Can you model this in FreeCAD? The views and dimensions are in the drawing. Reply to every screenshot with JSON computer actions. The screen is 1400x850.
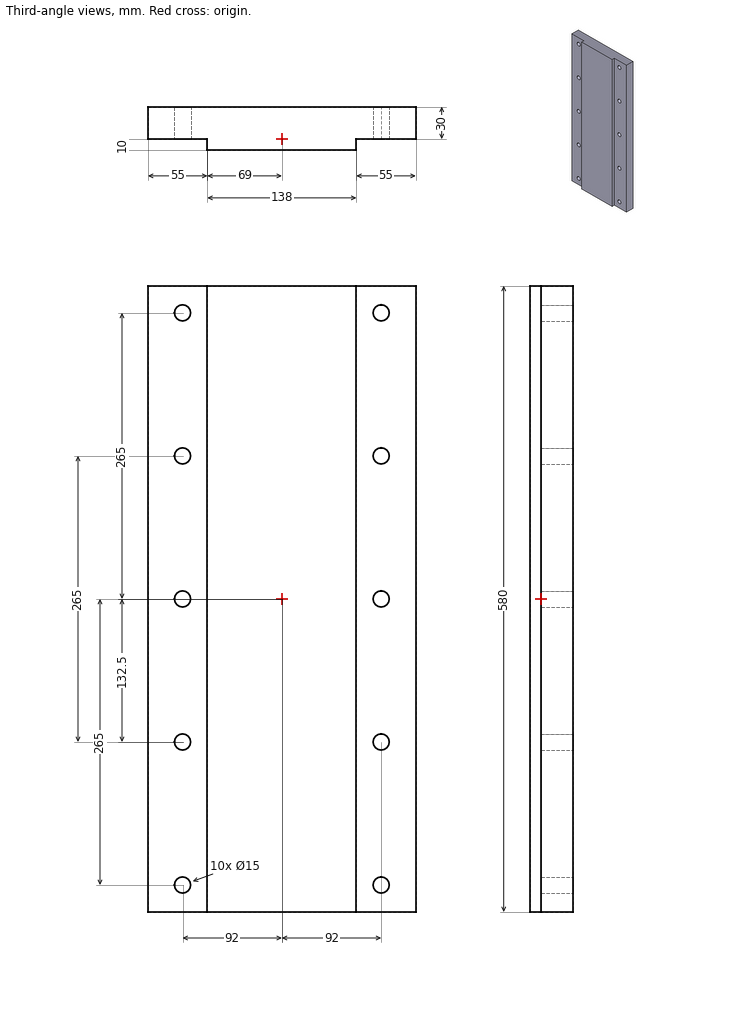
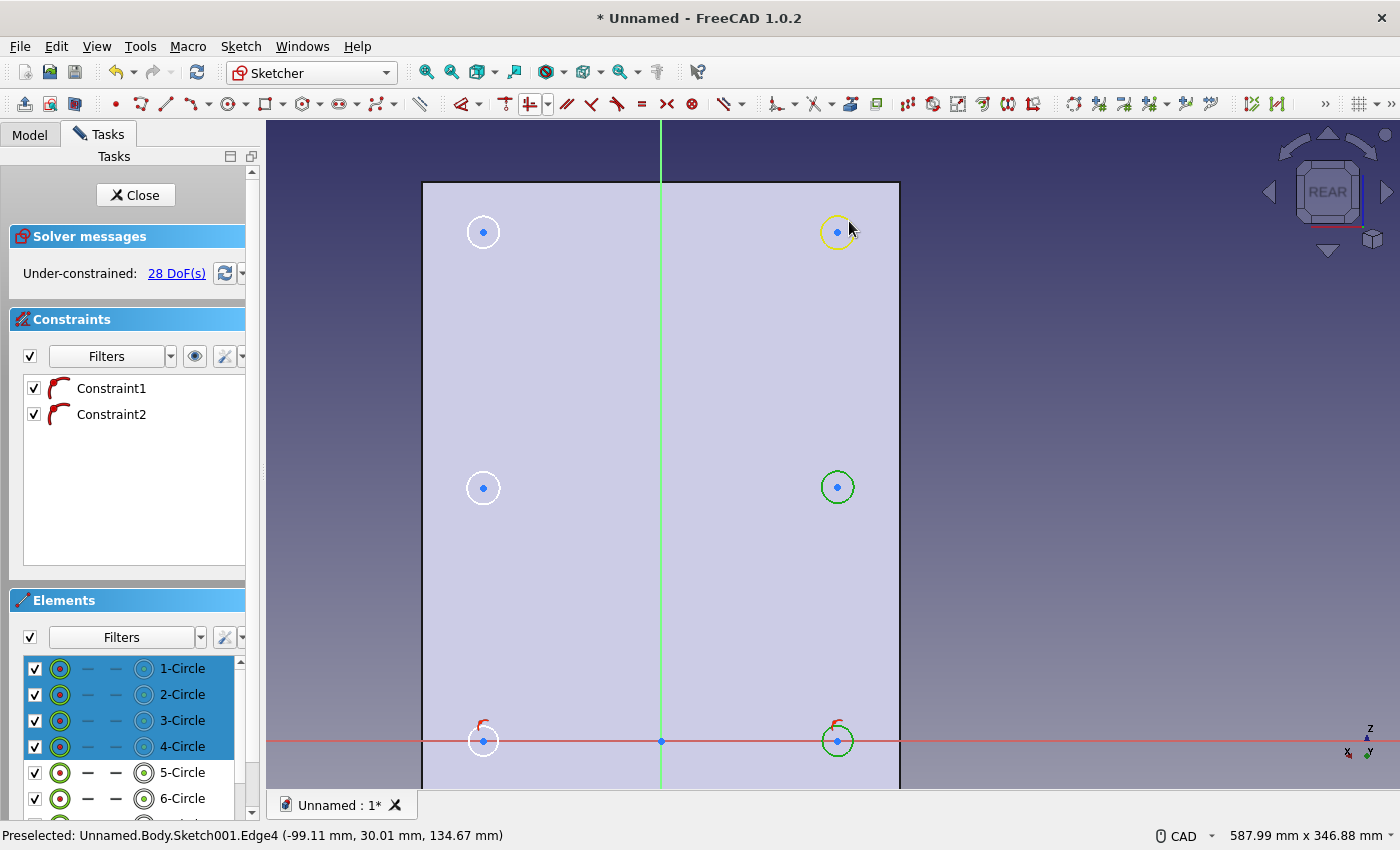
{"action": "left_click", "coordinate": [849, 221]}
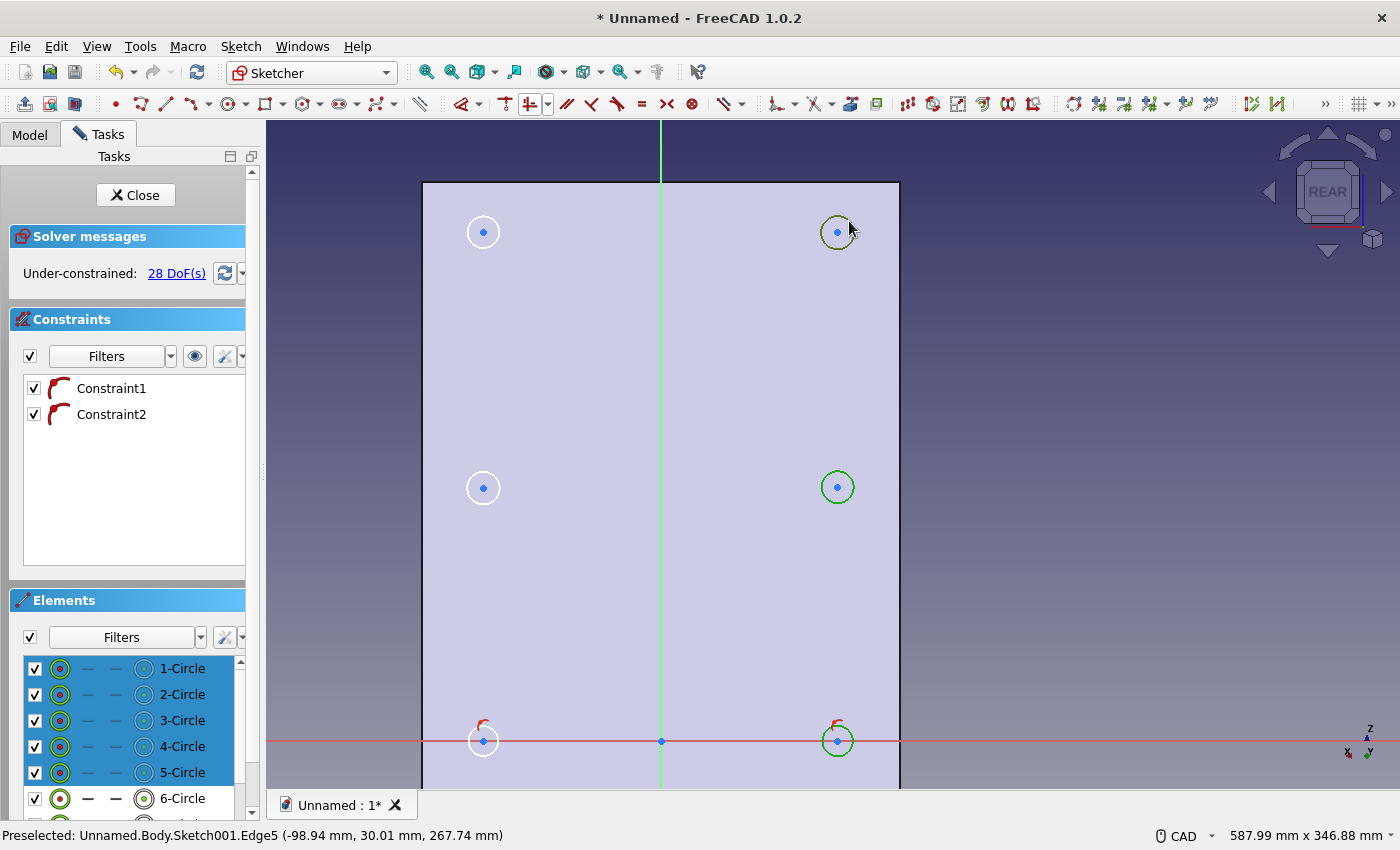
{"action": "scroll", "coordinate": [849, 221], "scroll_direction": "down", "scroll_amount": 4}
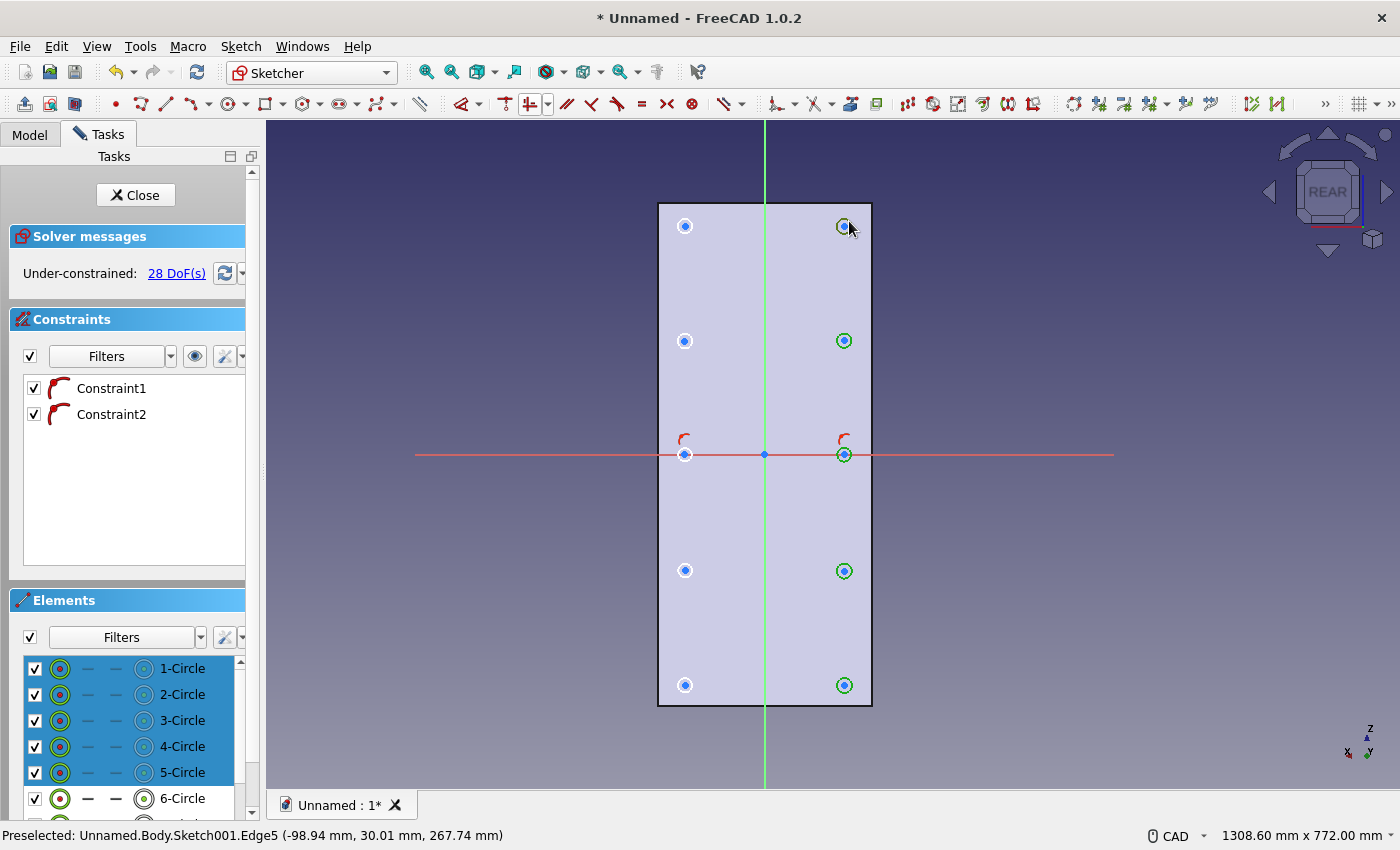
{"action": "scroll", "coordinate": [690, 566], "scroll_direction": "up", "scroll_amount": 4}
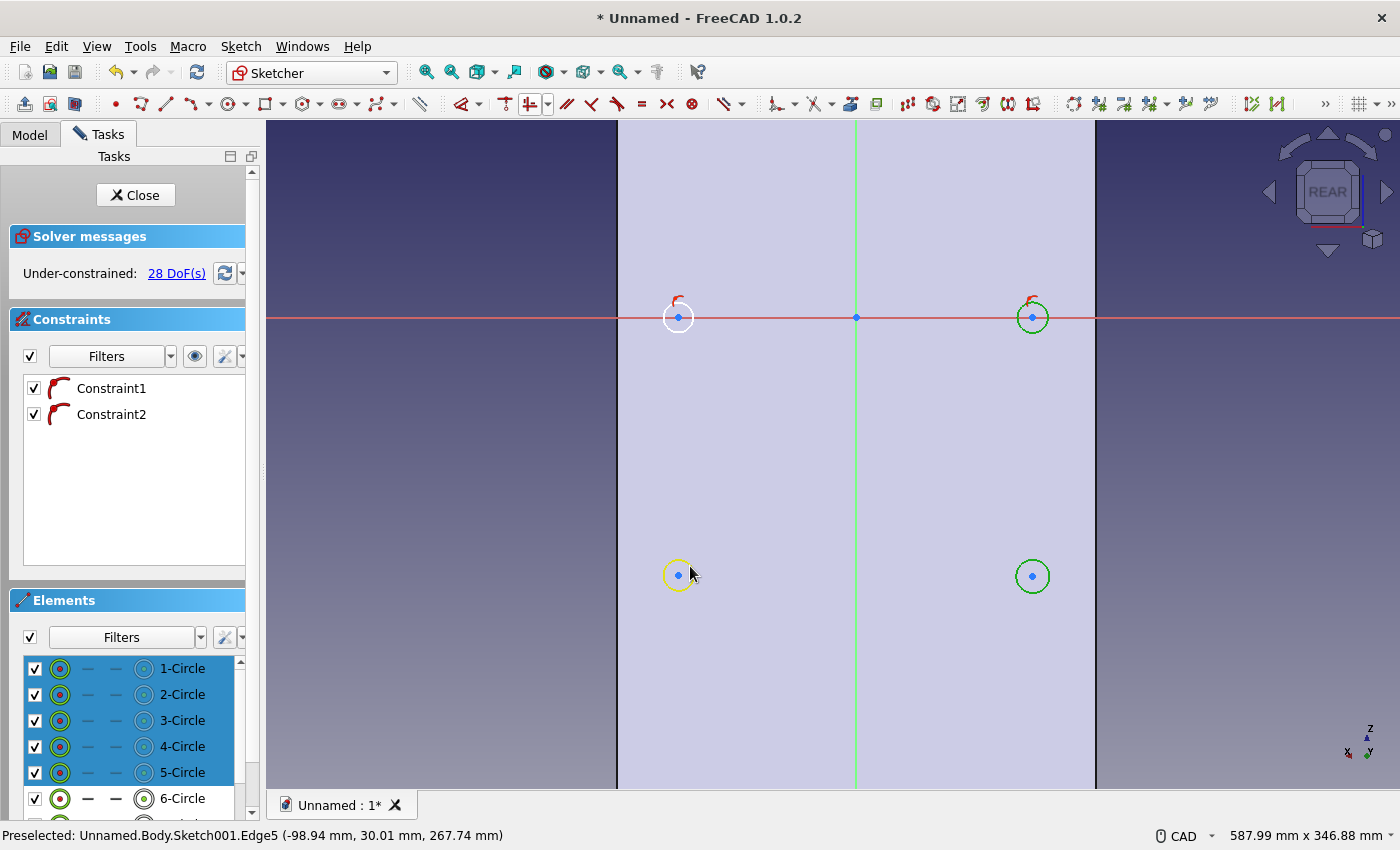
{"action": "left_click", "coordinate": [690, 565]}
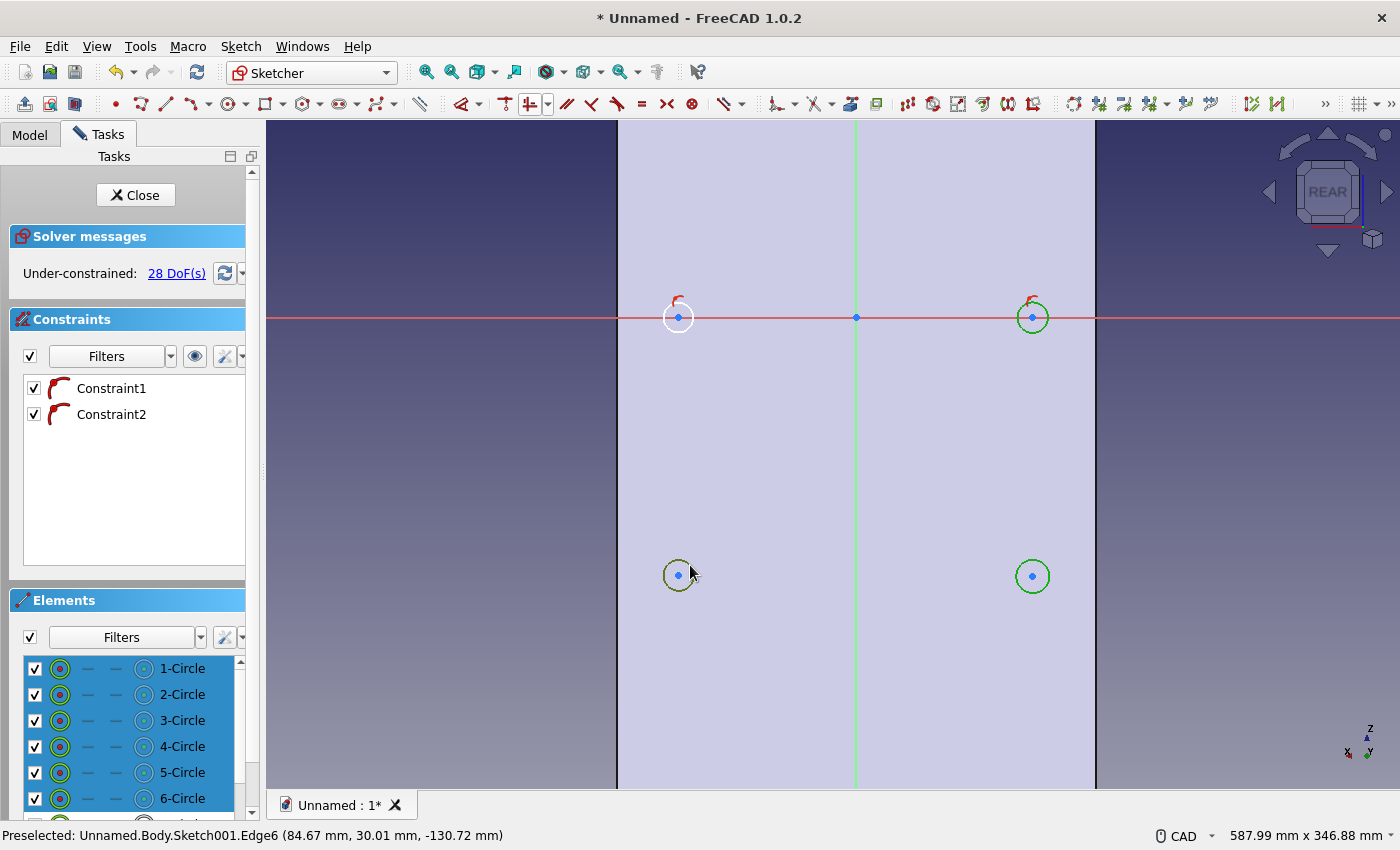
{"action": "scroll", "coordinate": [689, 307], "scroll_direction": "up", "scroll_amount": 2}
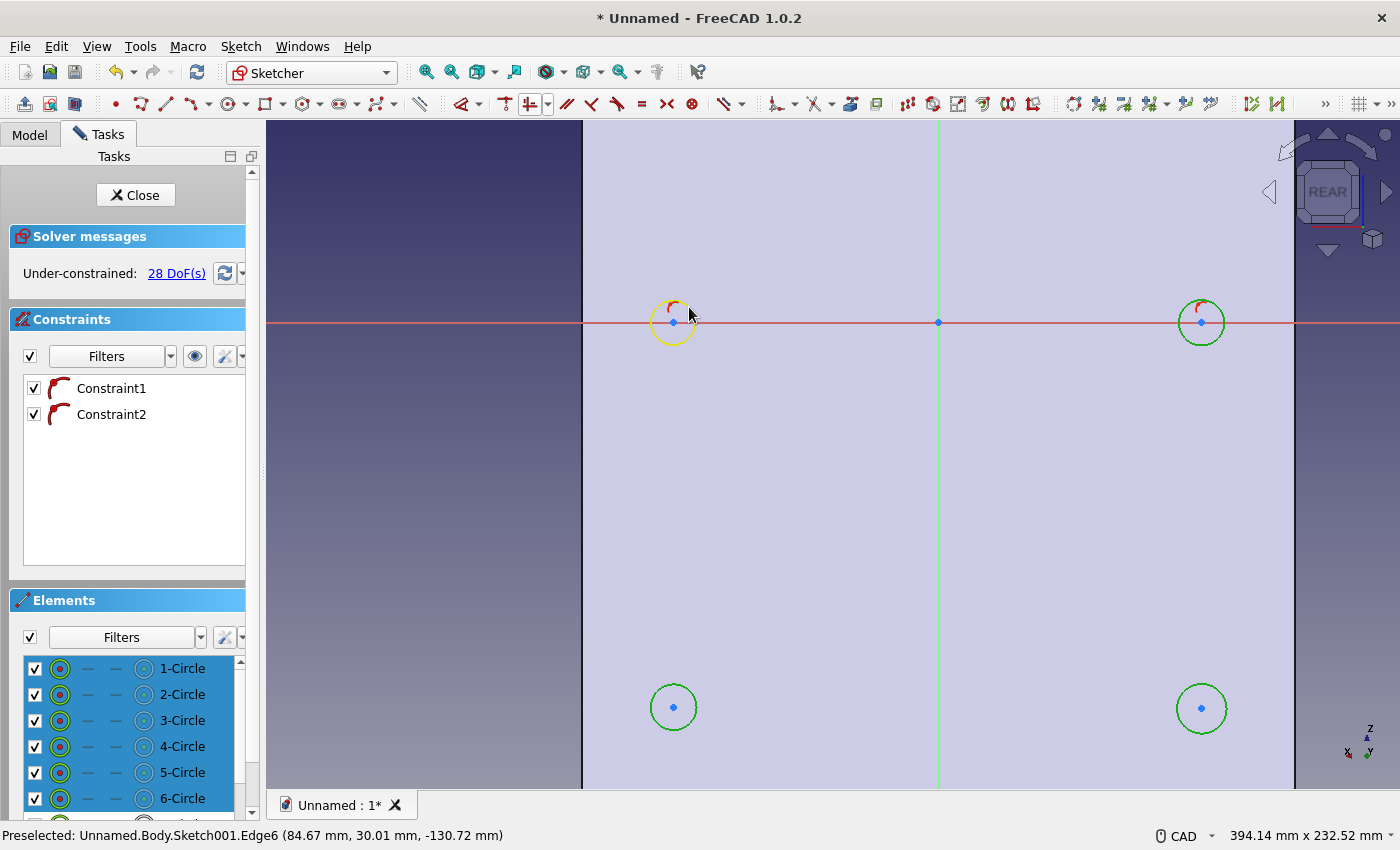
{"action": "left_click", "coordinate": [689, 307]}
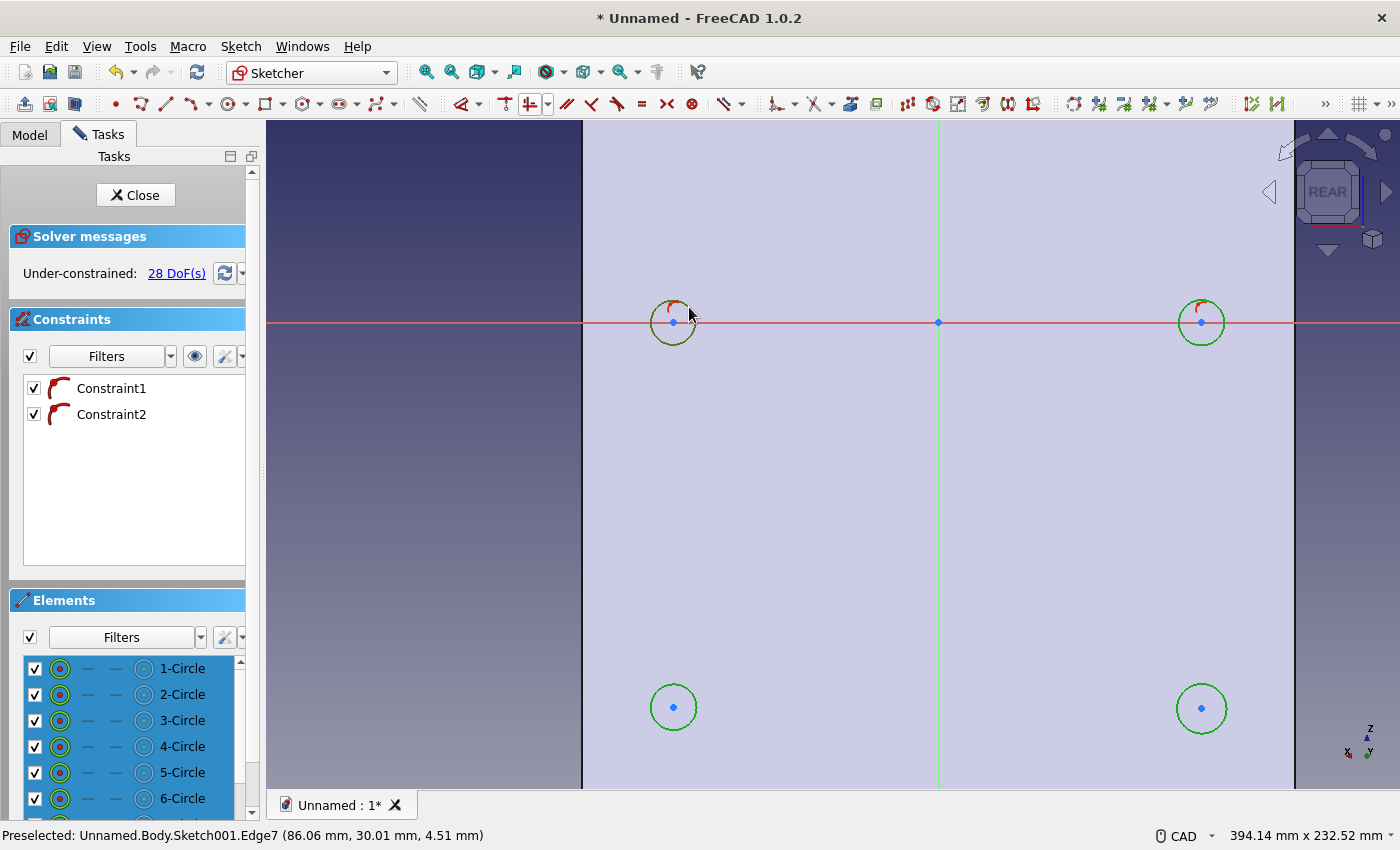
{"action": "scroll", "coordinate": [689, 511], "scroll_direction": "down", "scroll_amount": 6}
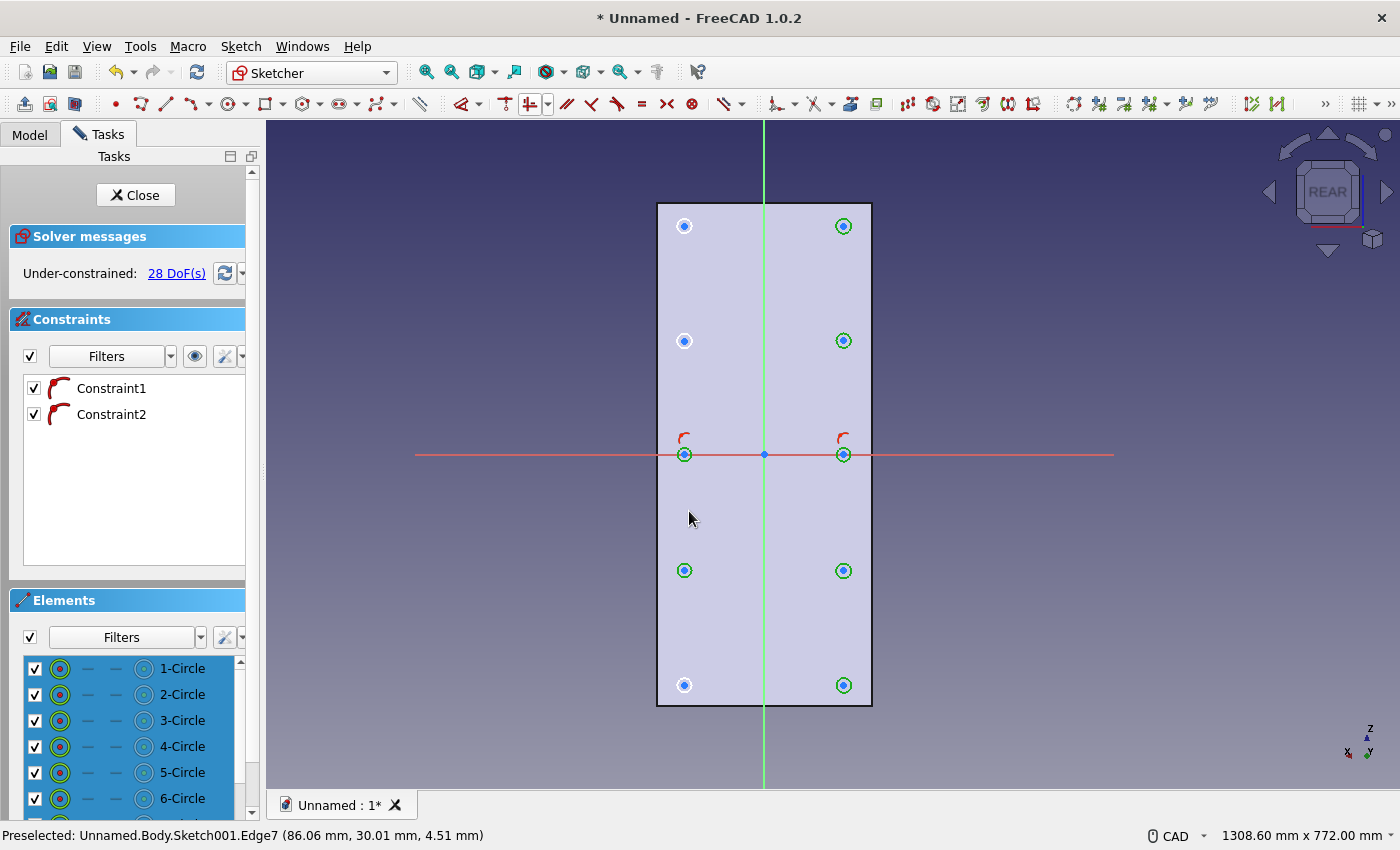
{"action": "scroll", "coordinate": [690, 336], "scroll_direction": "up", "scroll_amount": 4}